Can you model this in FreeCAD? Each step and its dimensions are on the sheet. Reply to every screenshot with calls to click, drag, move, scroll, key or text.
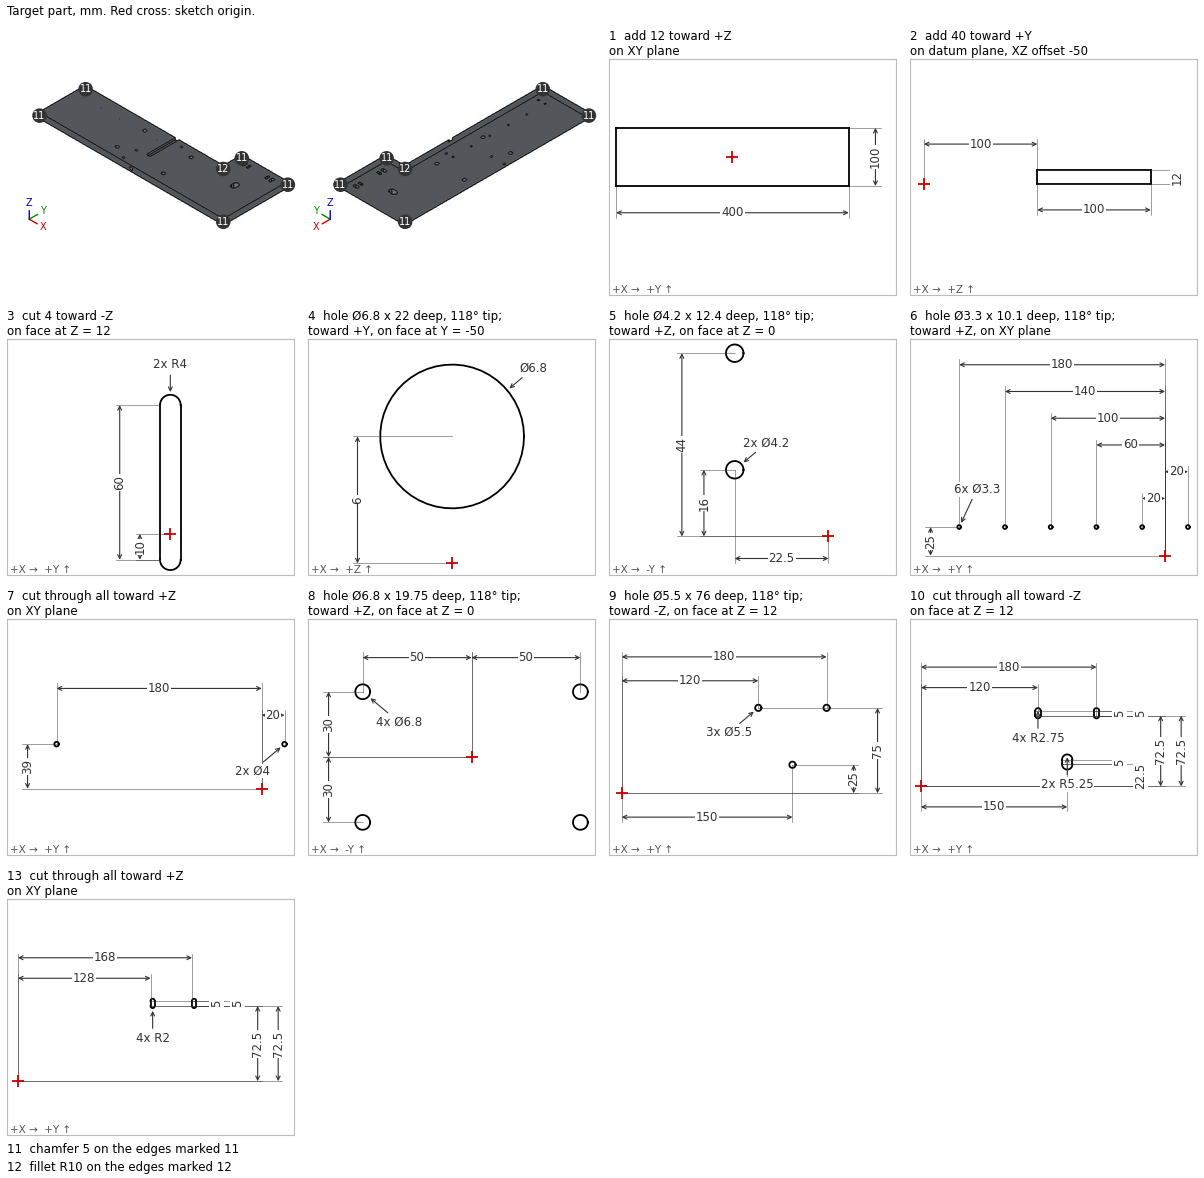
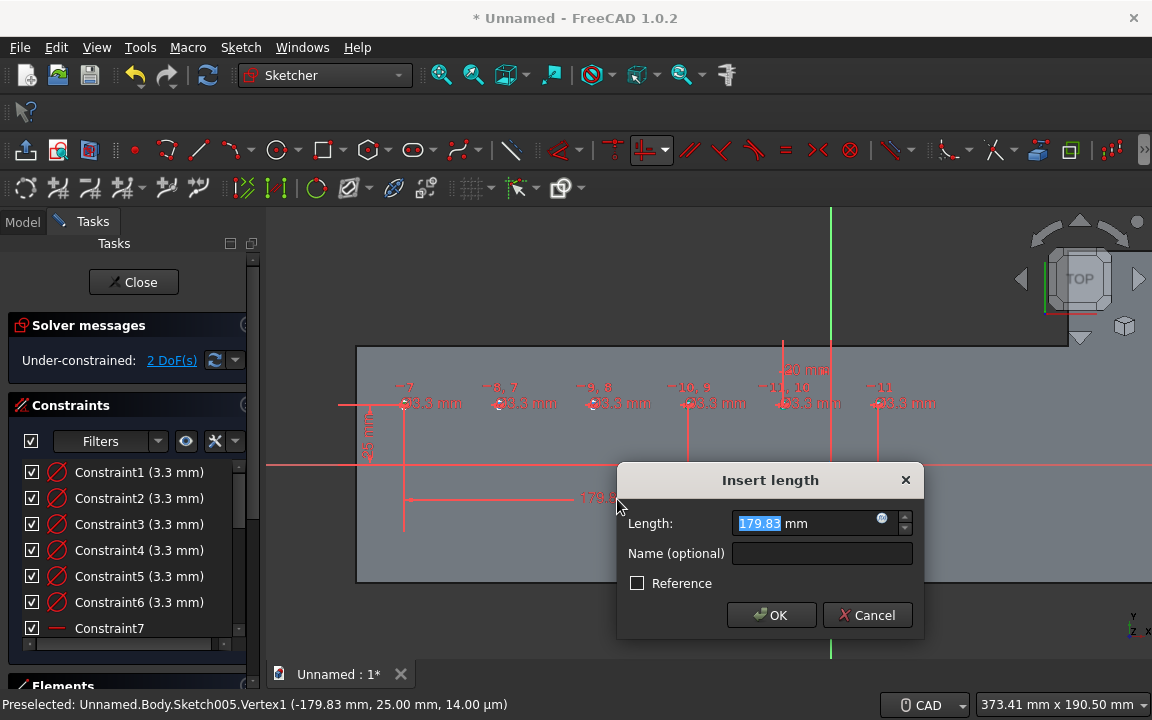
text(180)
key(Return)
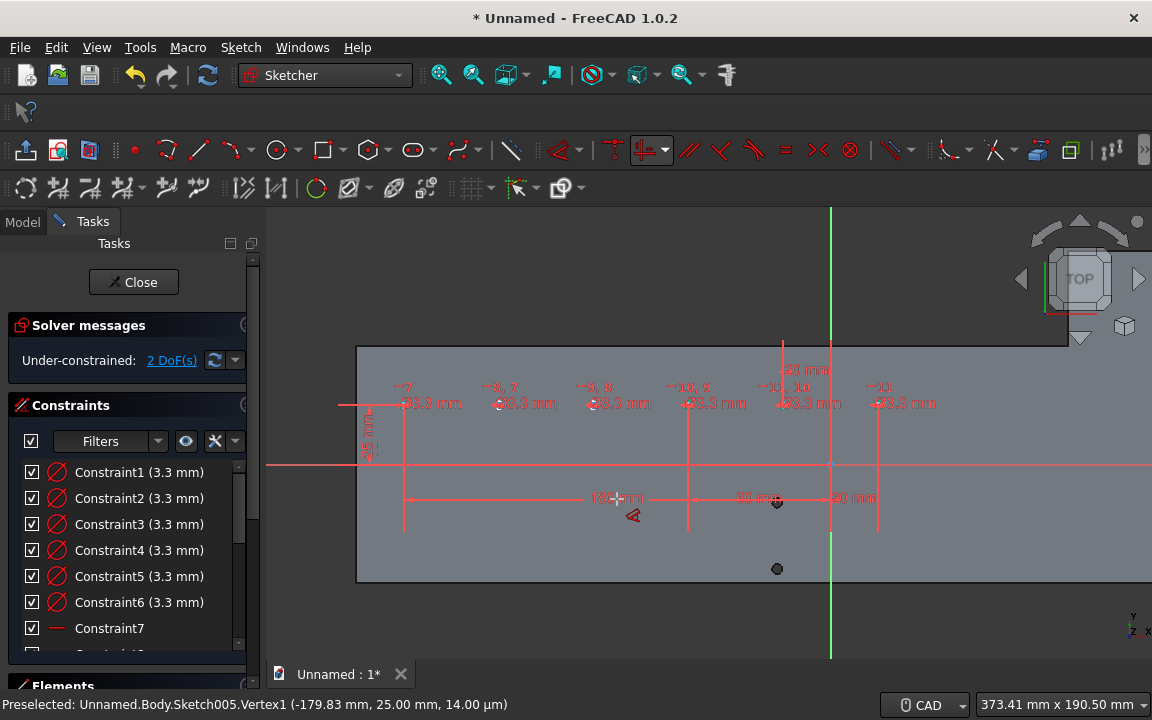
click(499, 405)
click(665, 371)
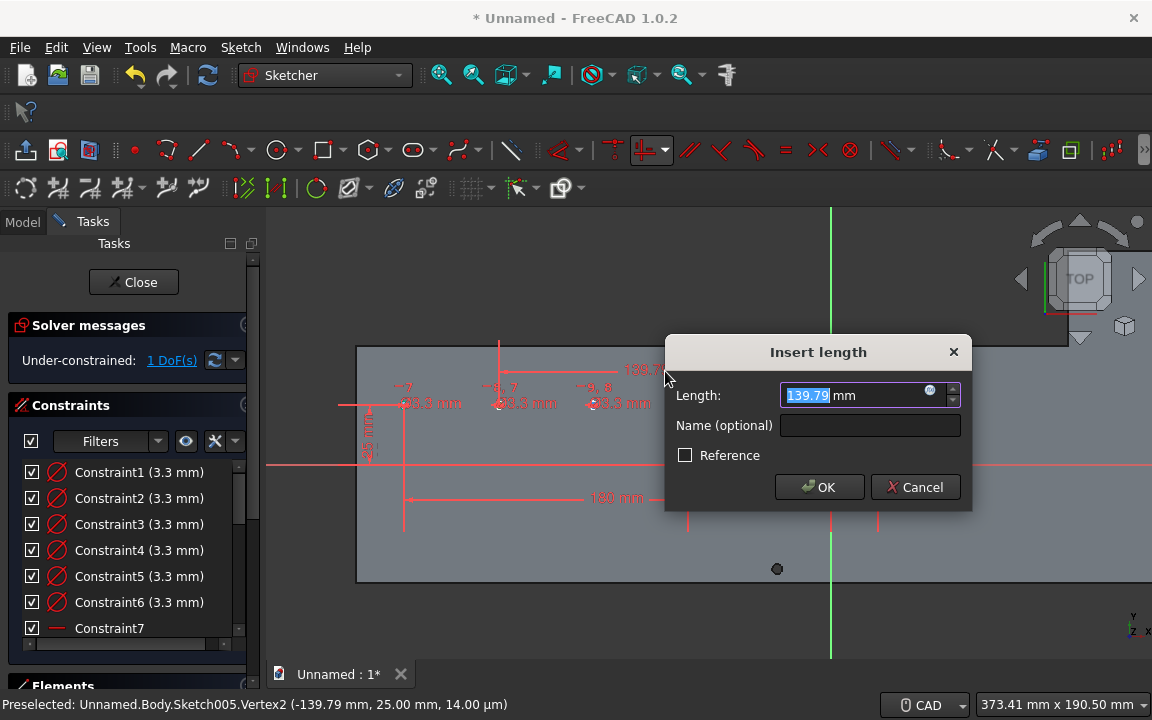
text(140)
key(Return)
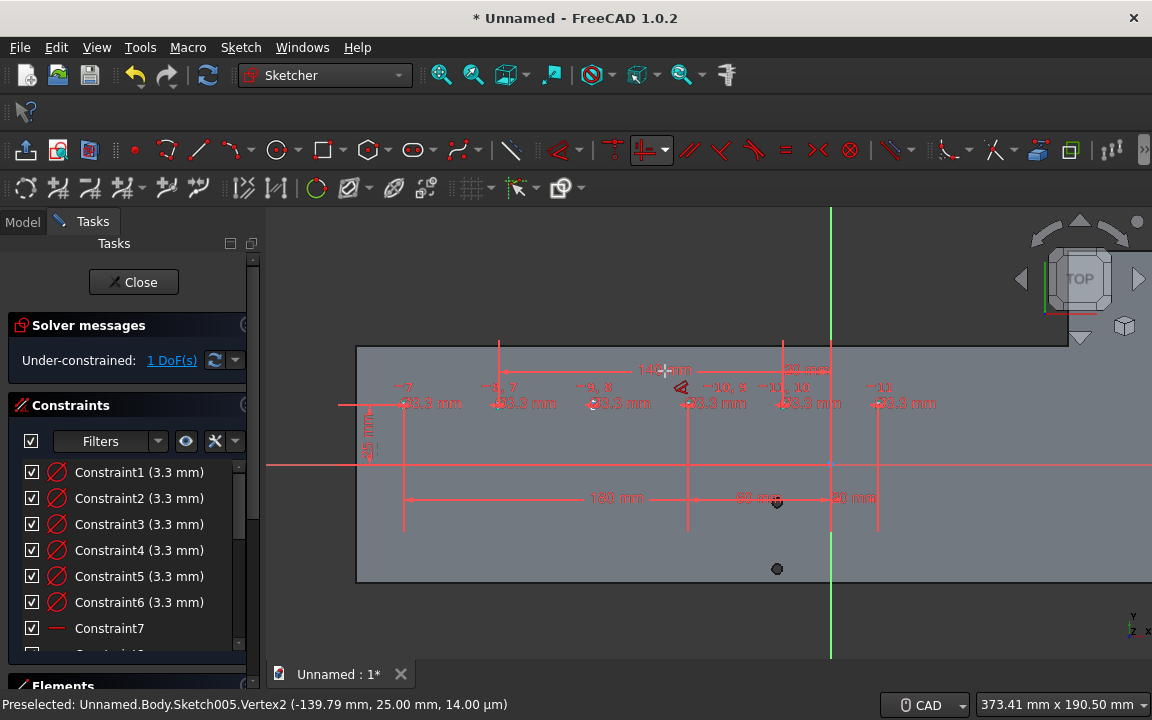
click(593, 405)
click(712, 523)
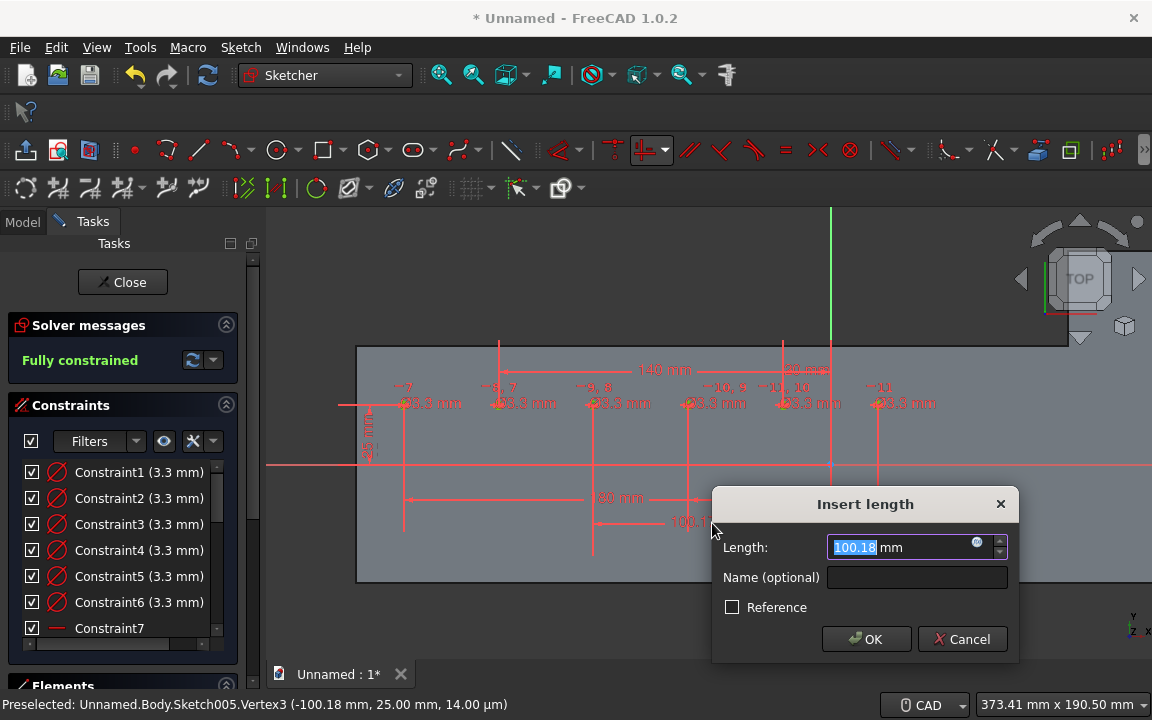
text(100)
key(Return)
key(Escape)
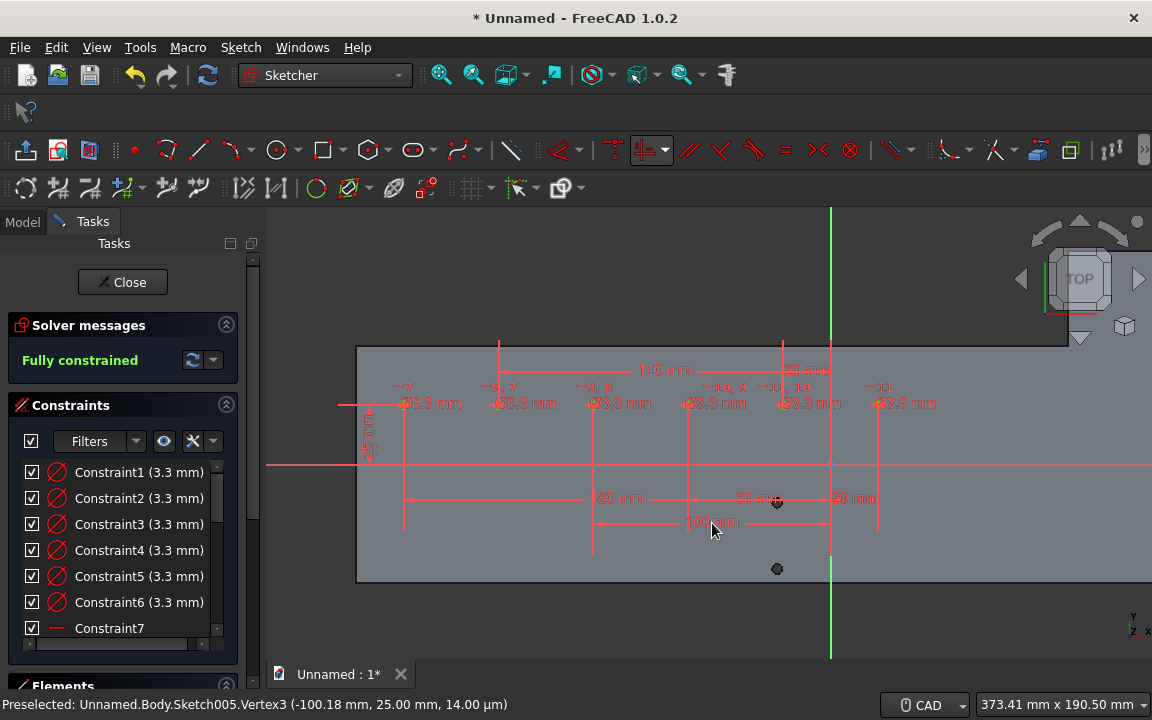
click(123, 282)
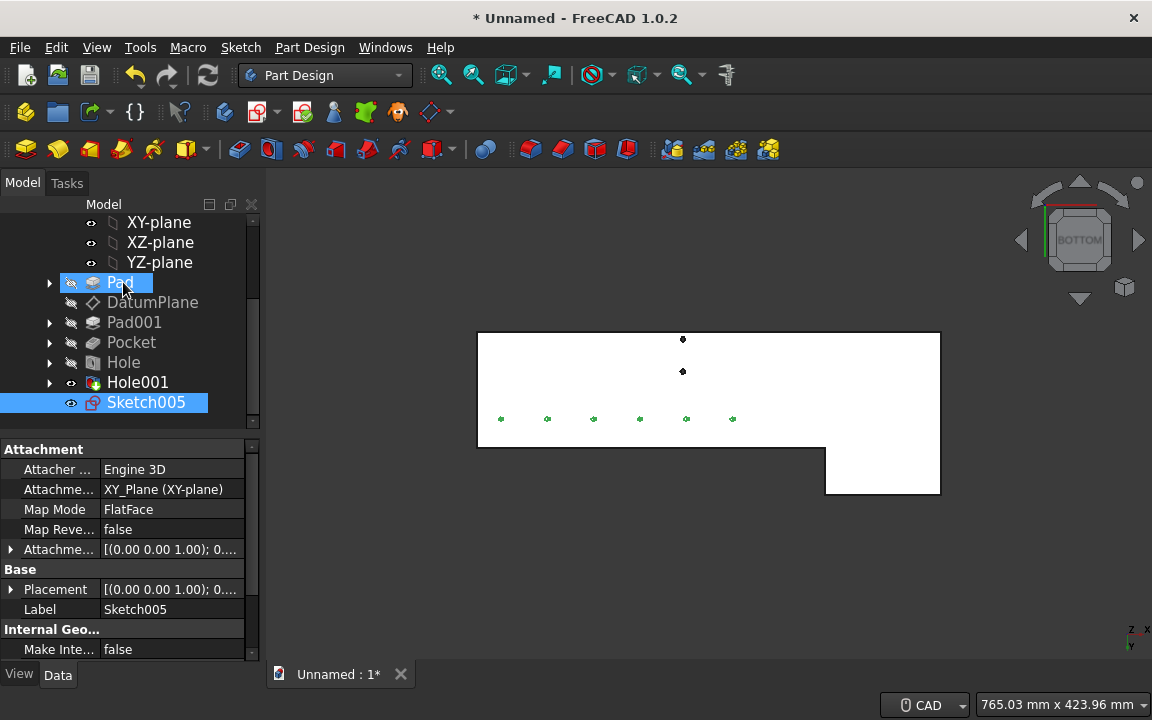
click(272, 150)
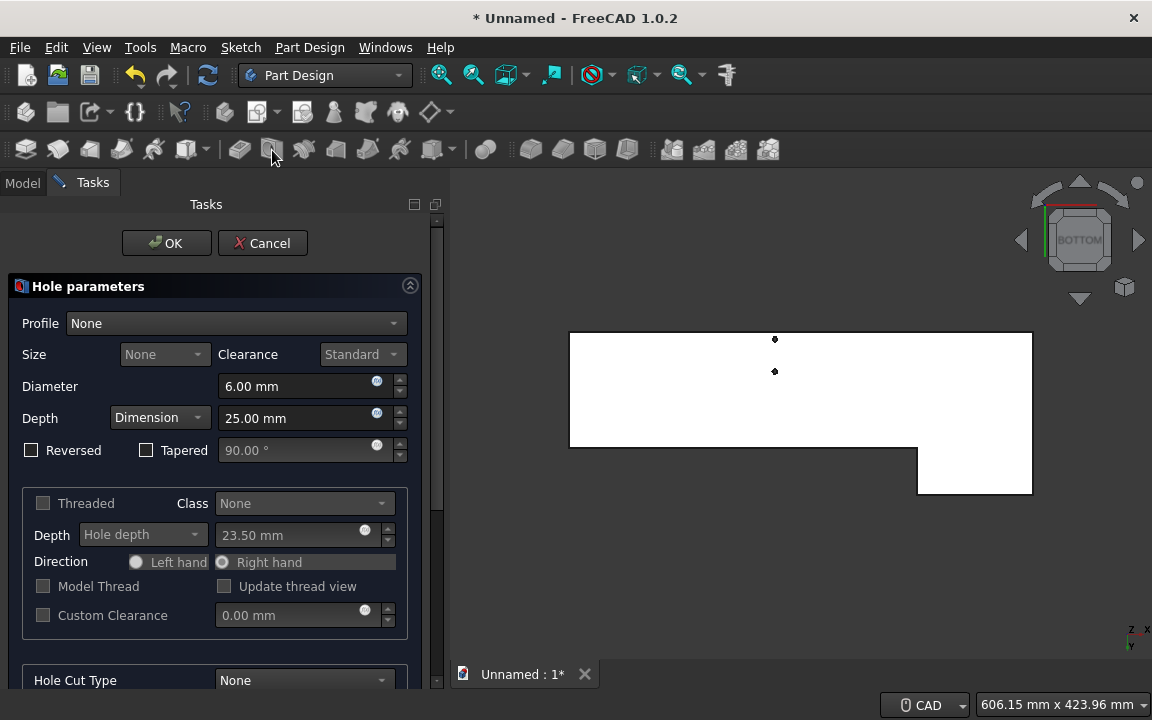
triple_click(305, 386)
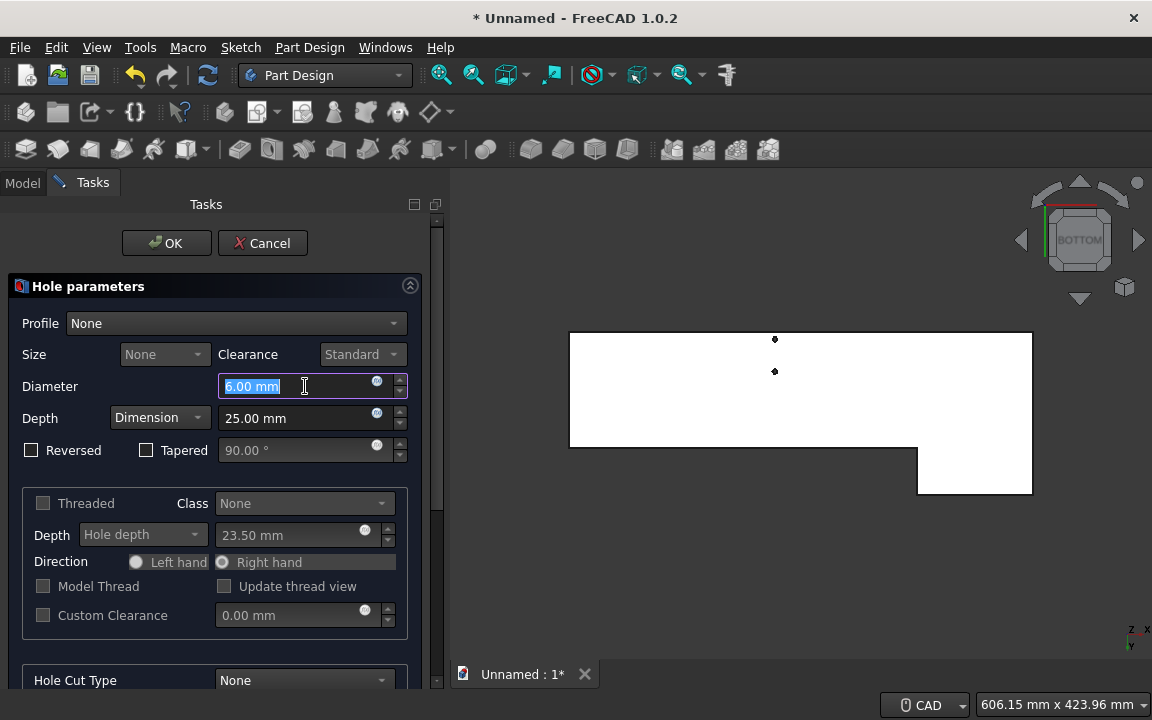
text(3.3)
key(Tab)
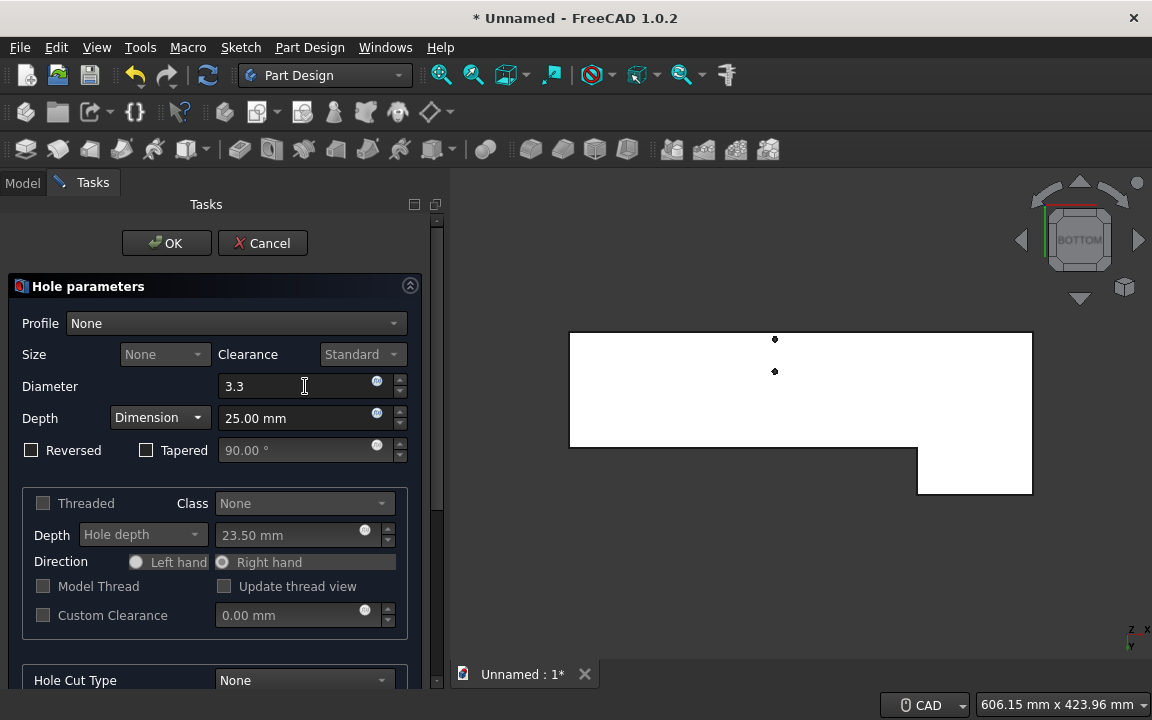
triple_click(305, 418)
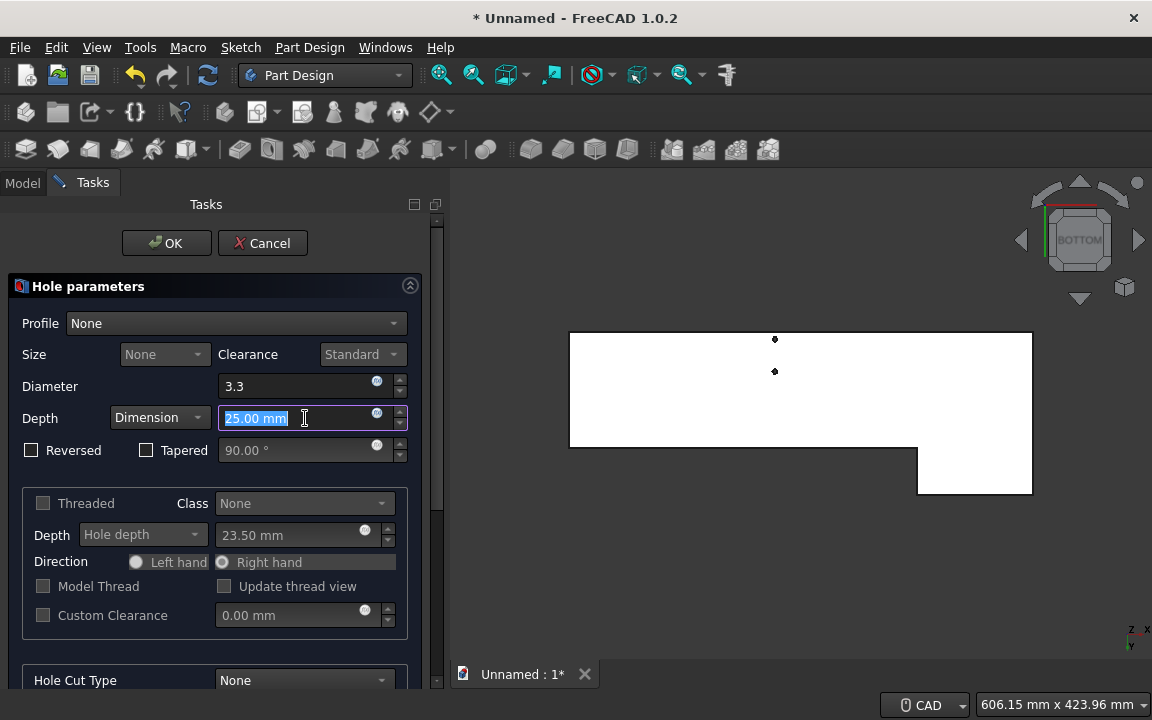
text(10.1)
key(Tab)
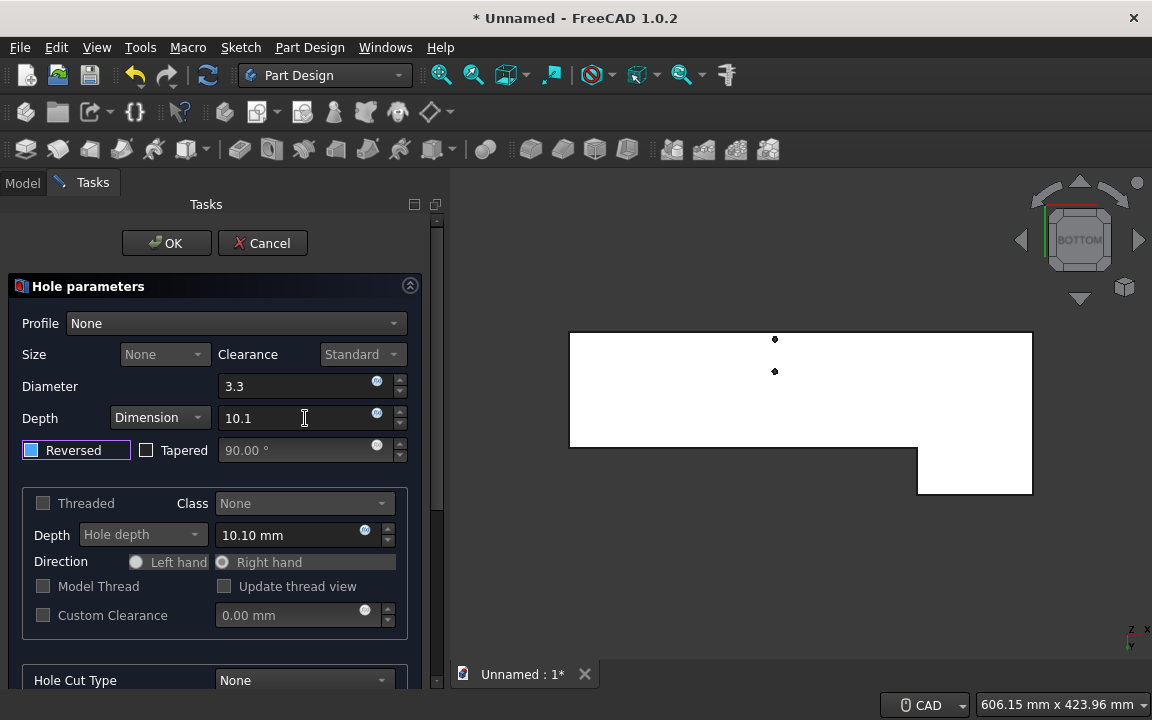
click(30, 450)